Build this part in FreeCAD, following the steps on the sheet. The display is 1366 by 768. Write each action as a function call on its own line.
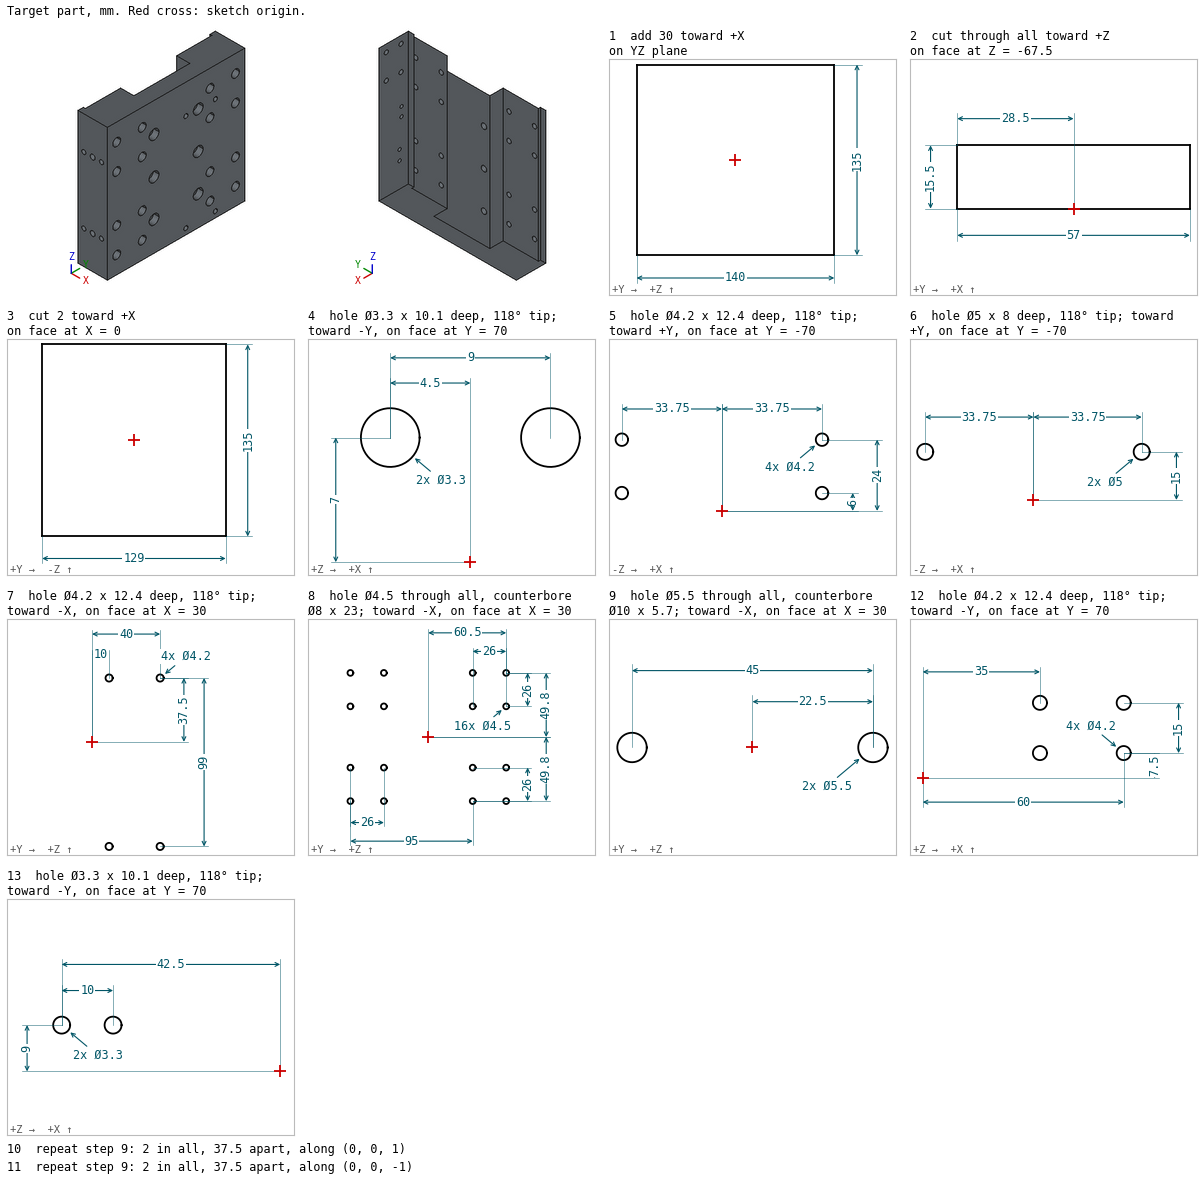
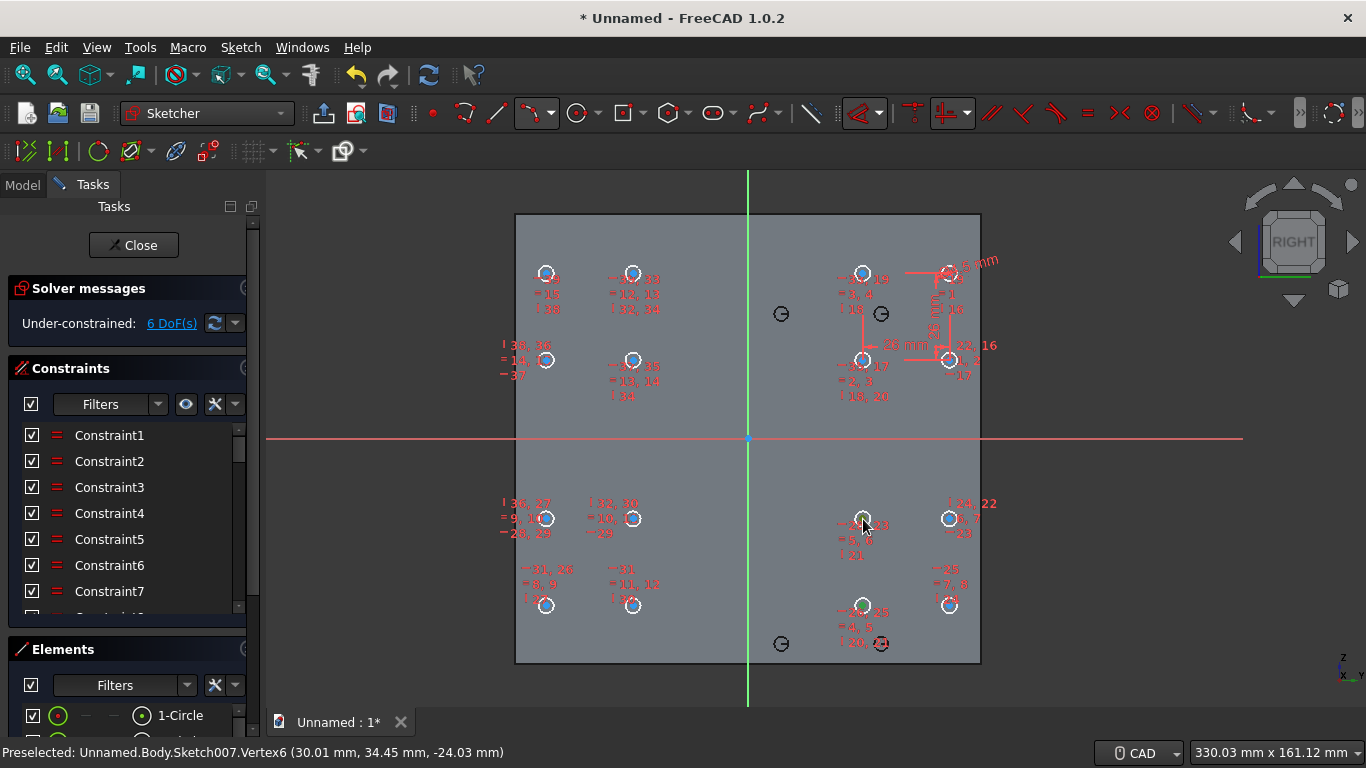
key(i)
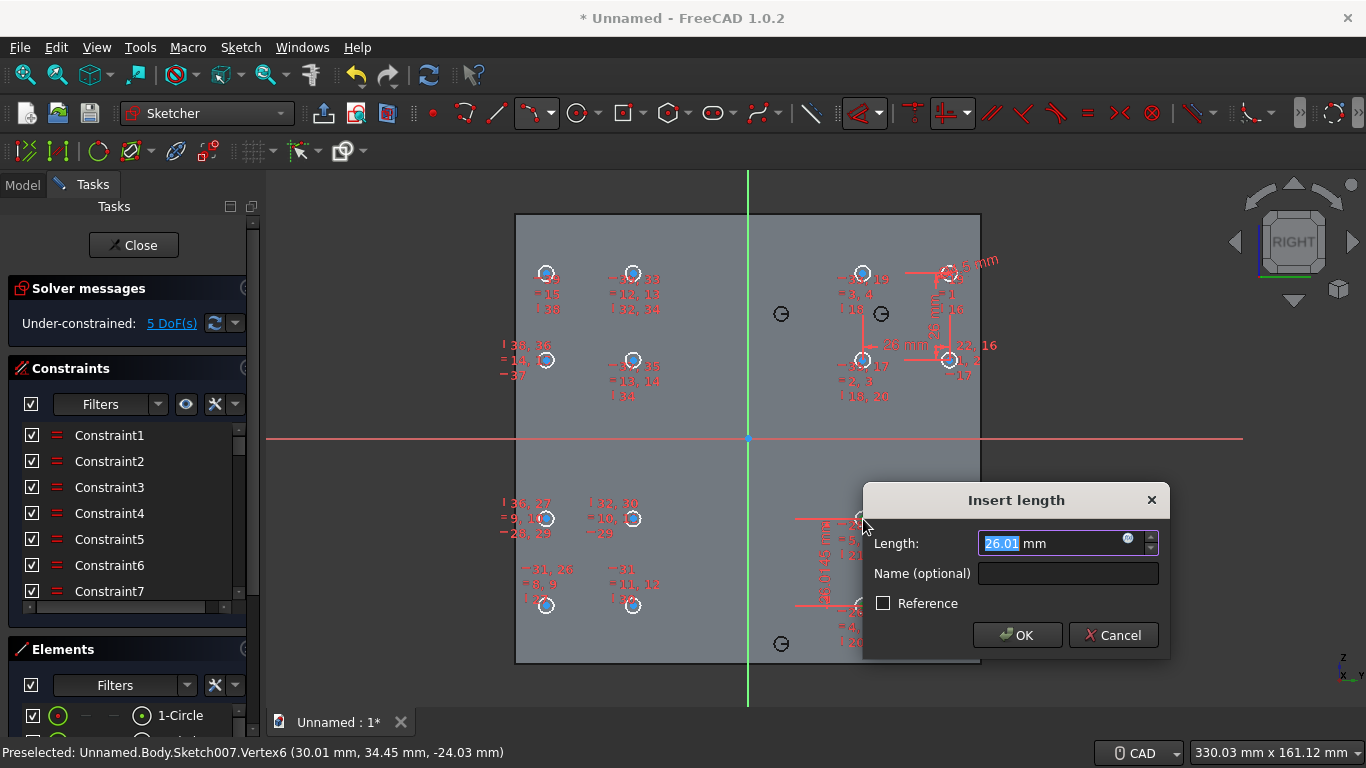
text(26)
key(Return)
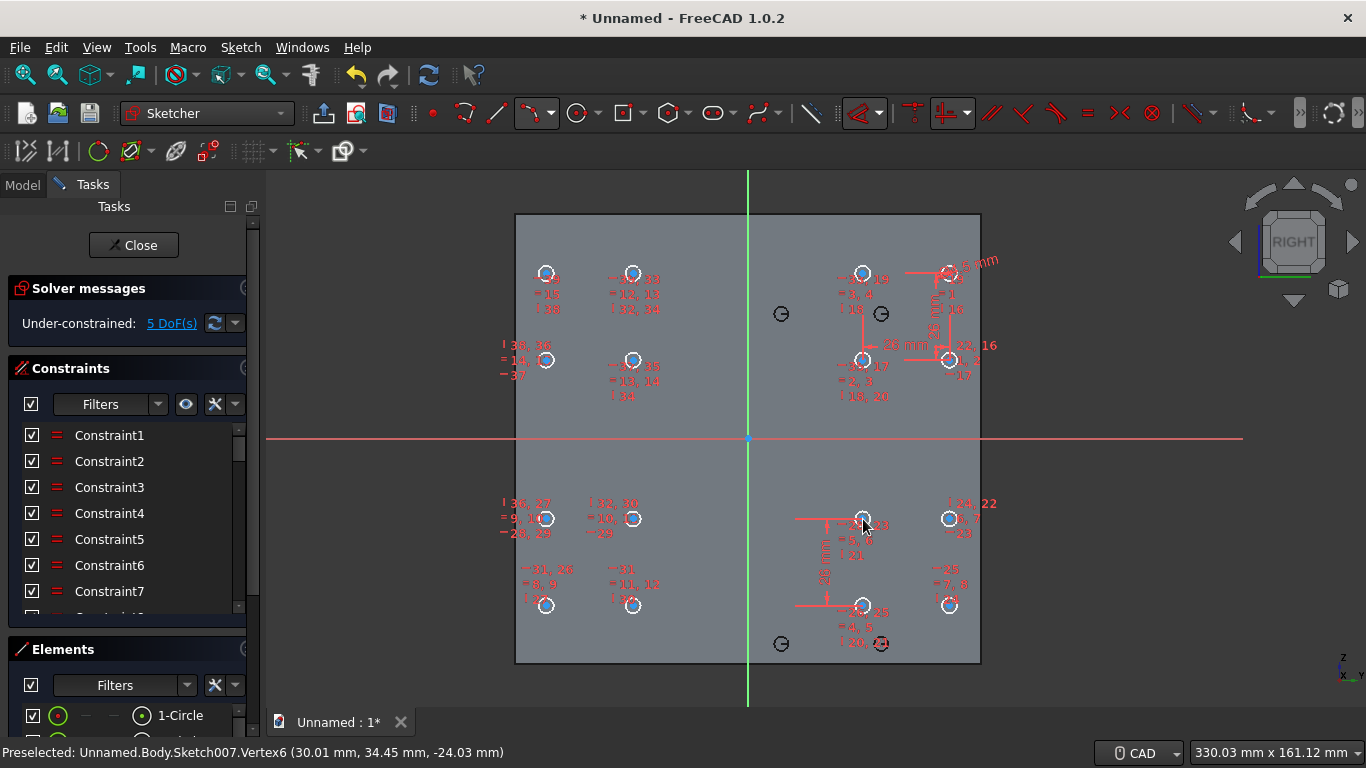
click(863, 606)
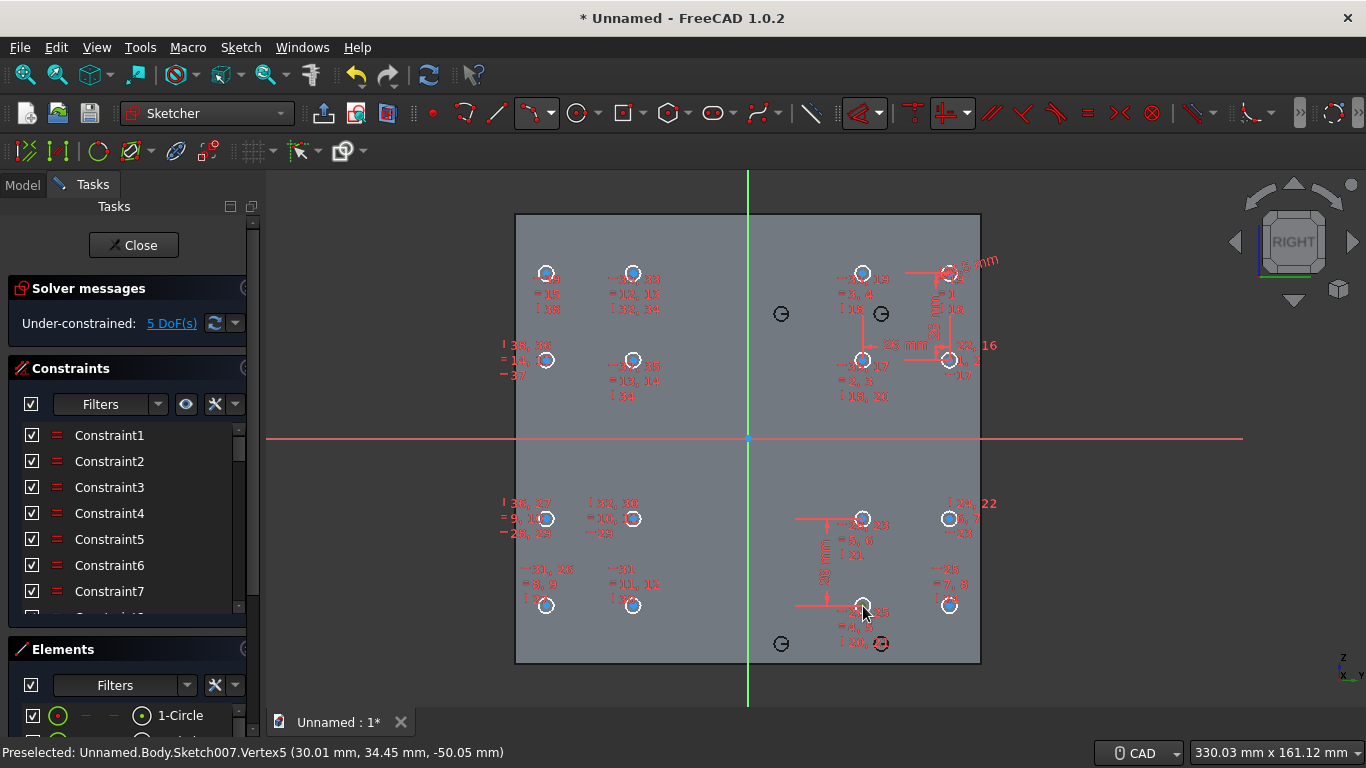
click(546, 606)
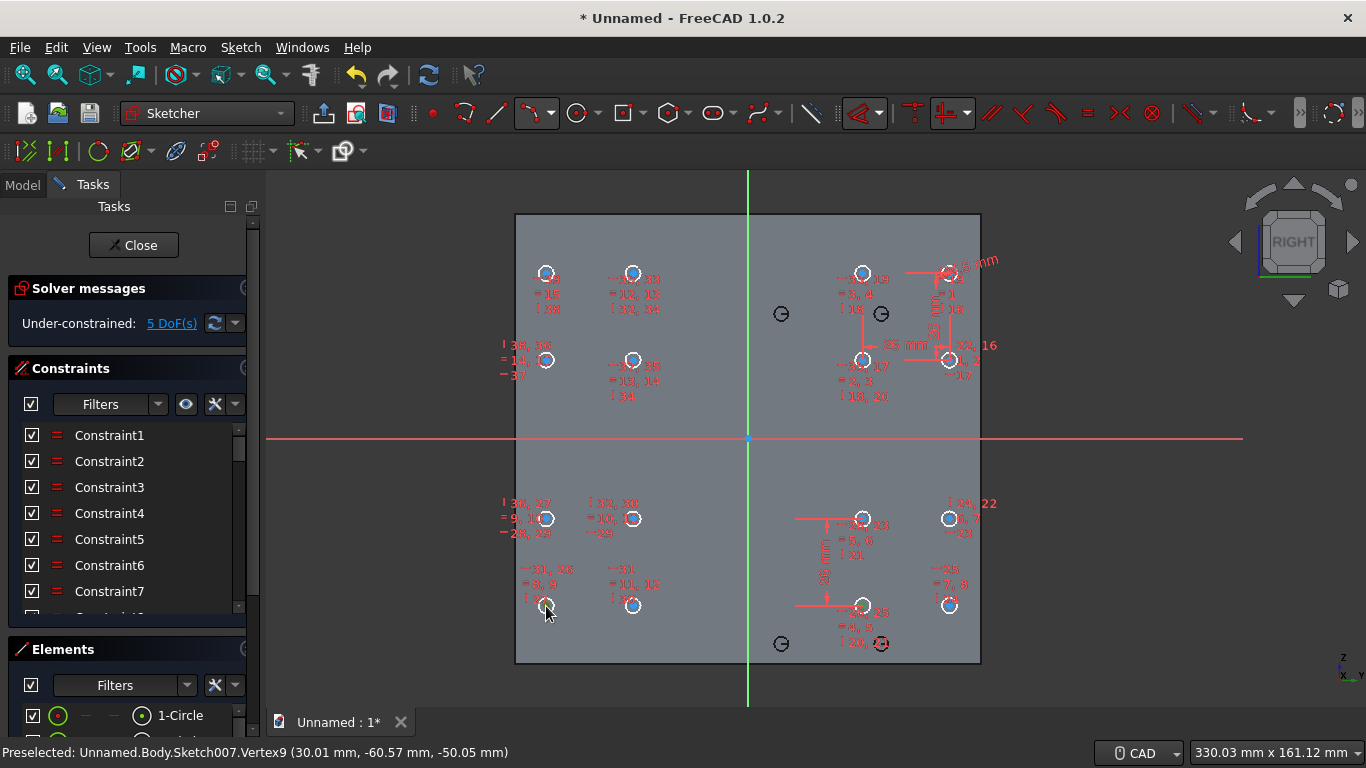
click(882, 114)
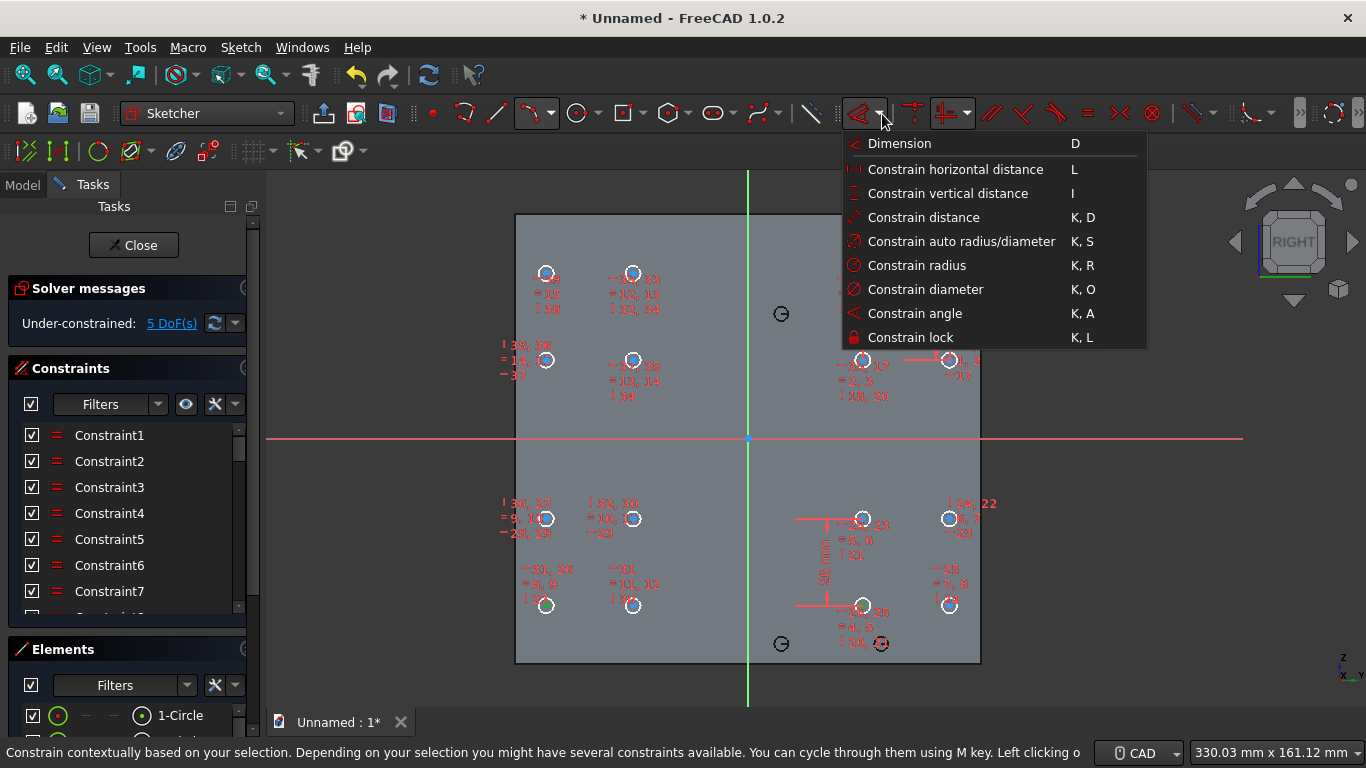
click(995, 169)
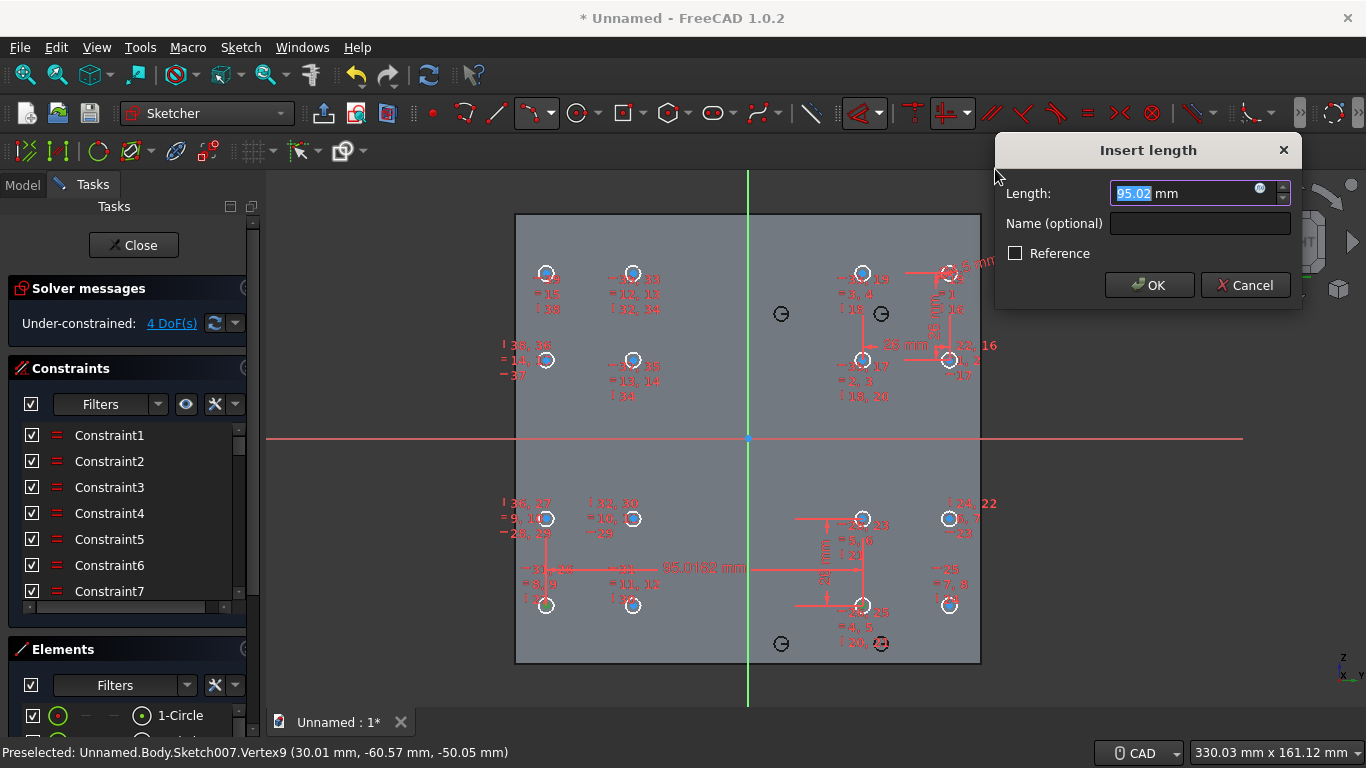
text(95)
key(Return)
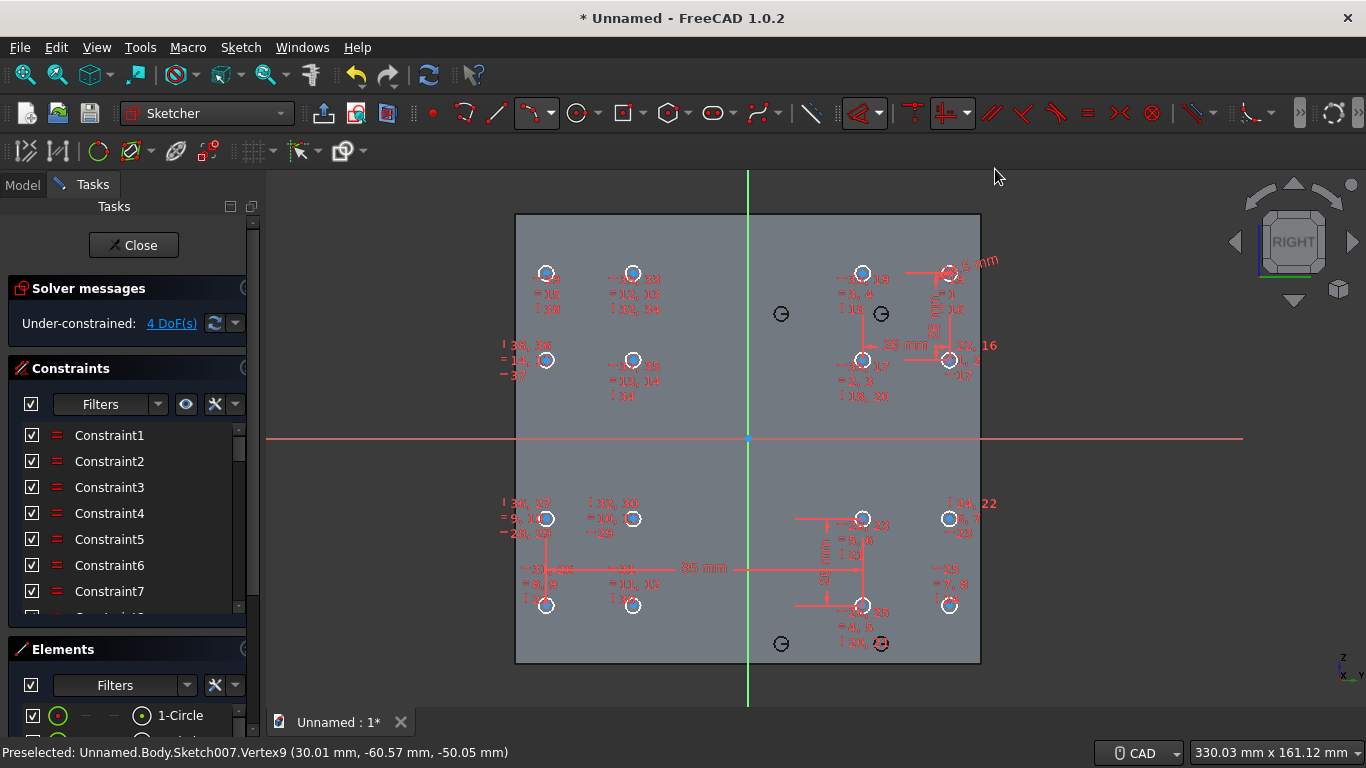
click(546, 519)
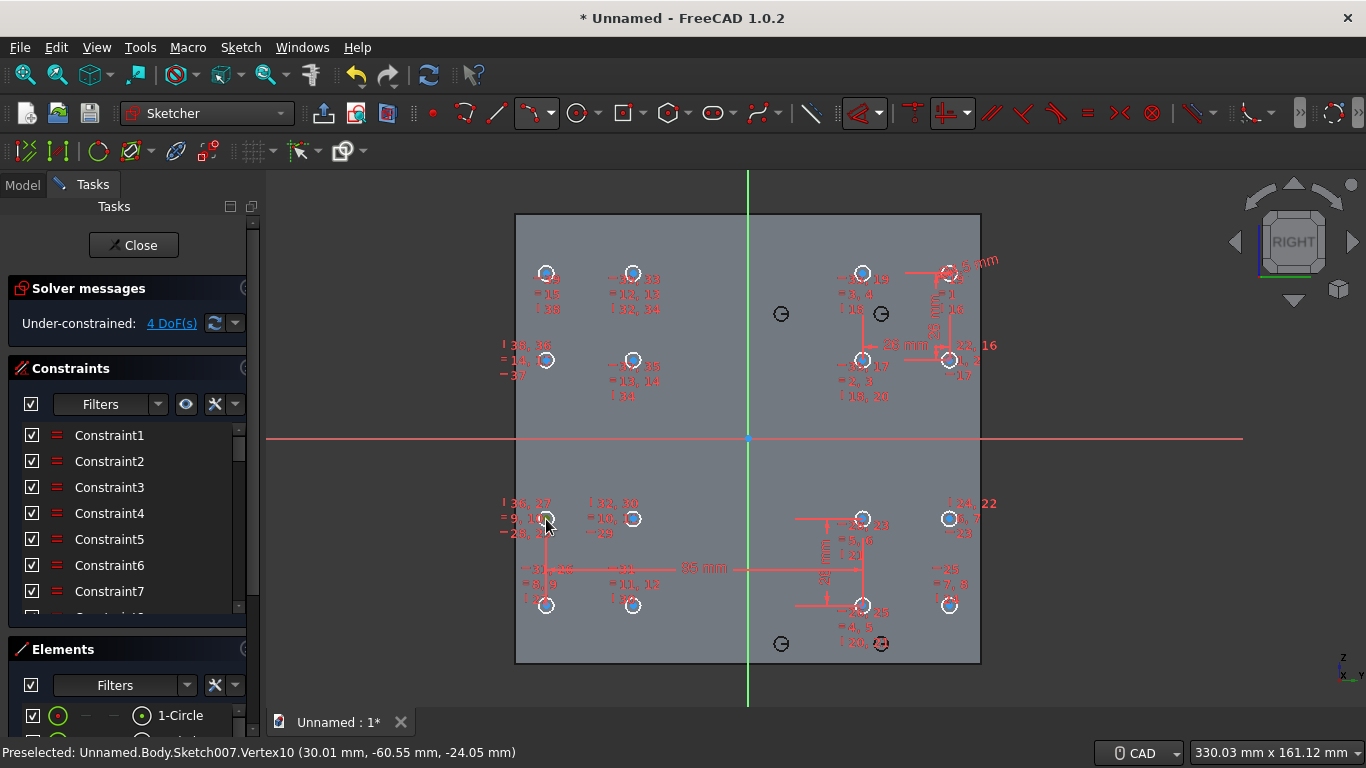
click(633, 519)